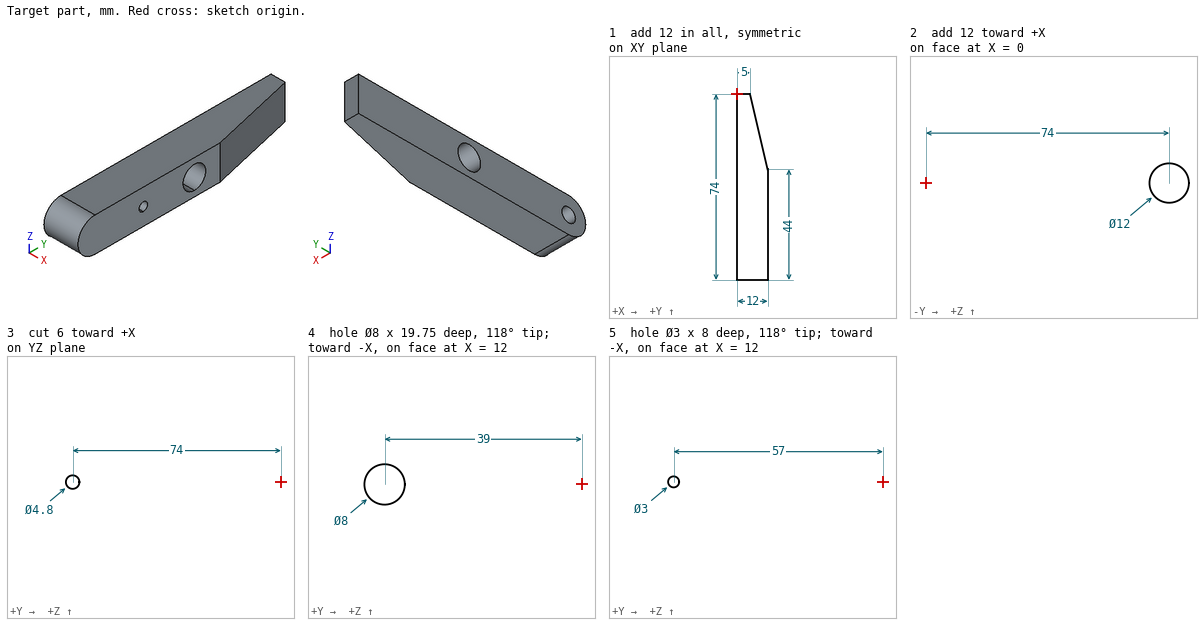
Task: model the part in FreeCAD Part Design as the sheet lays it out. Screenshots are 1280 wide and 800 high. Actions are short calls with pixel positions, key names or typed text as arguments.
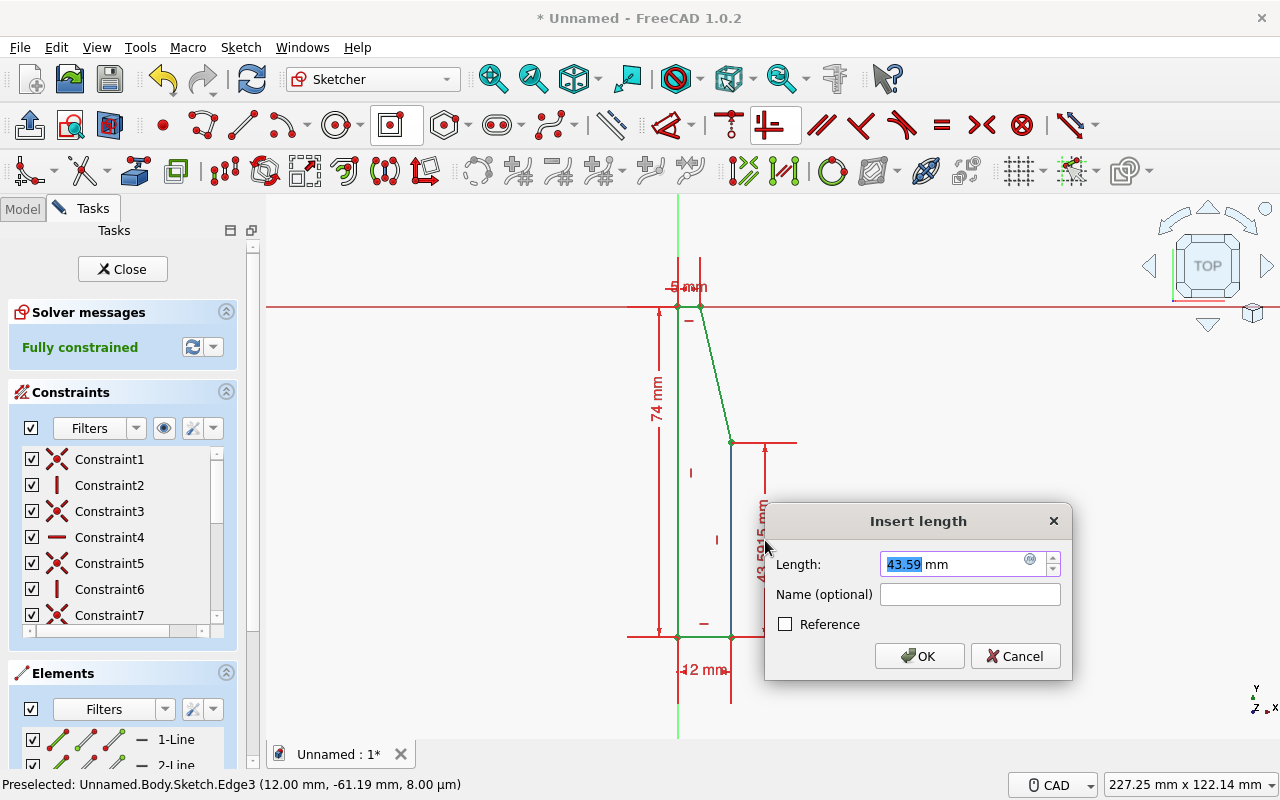
text(44)
key(Return)
key(Escape)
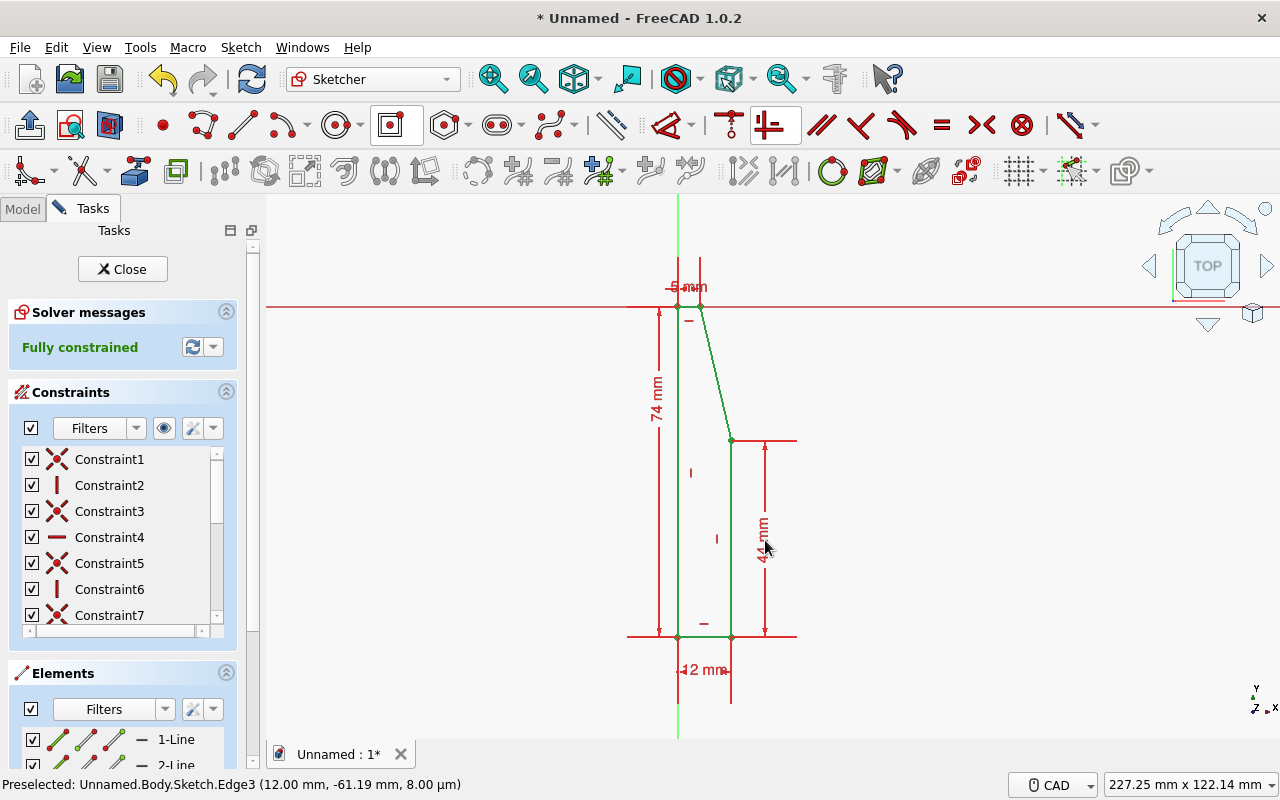
click(123, 269)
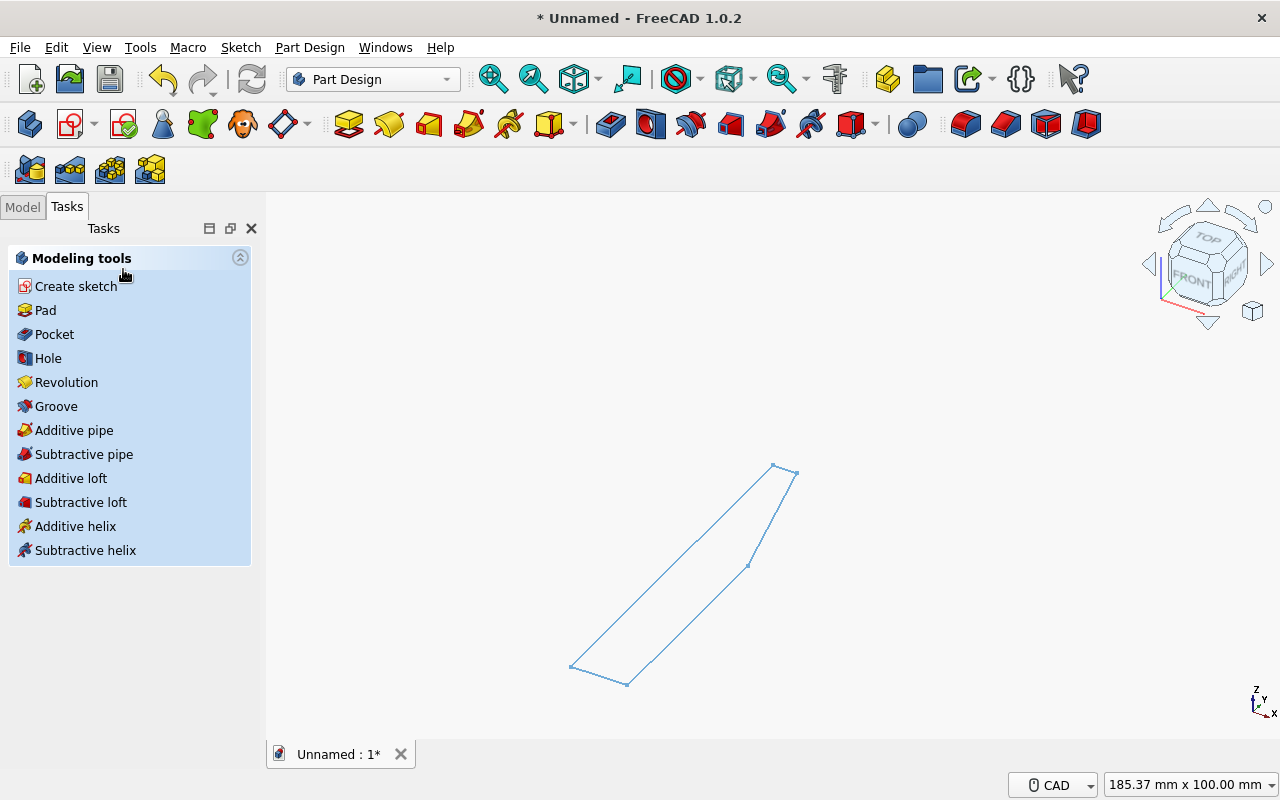
click(350, 124)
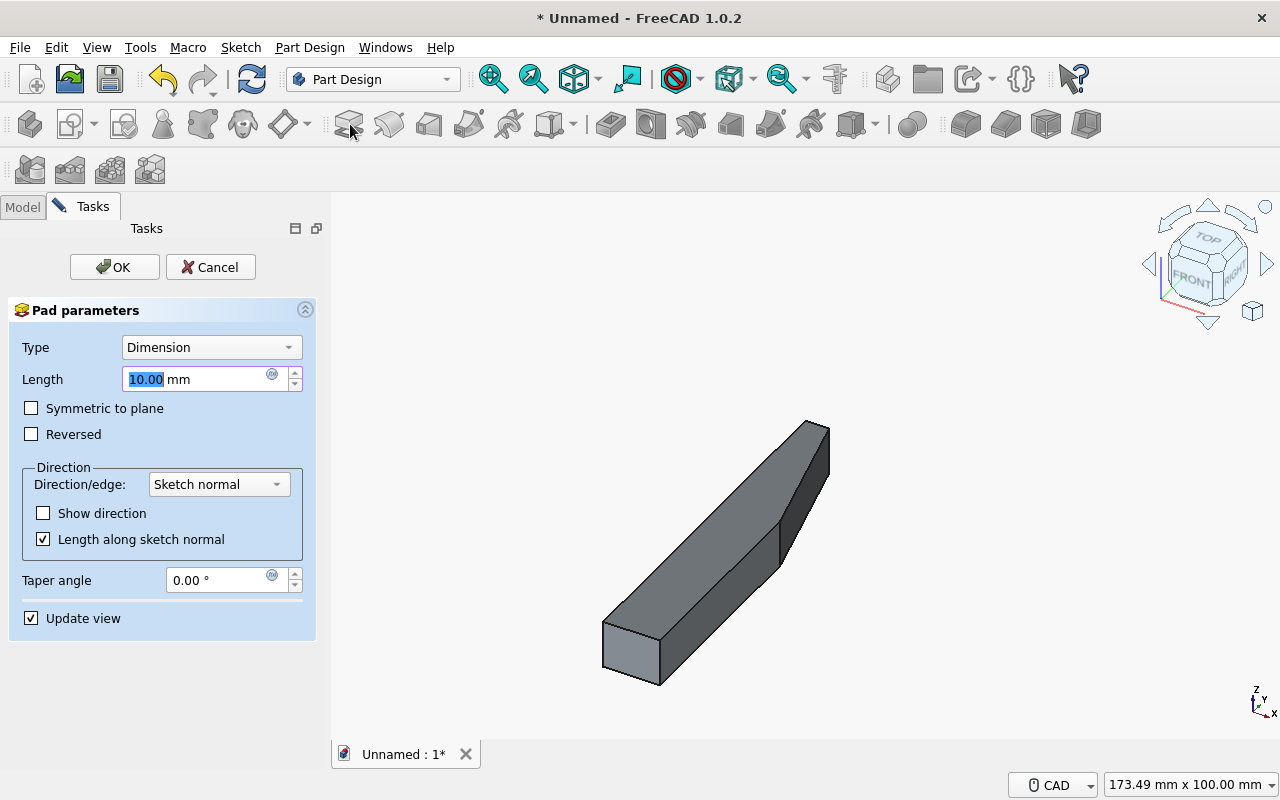
text(12)
key(Tab)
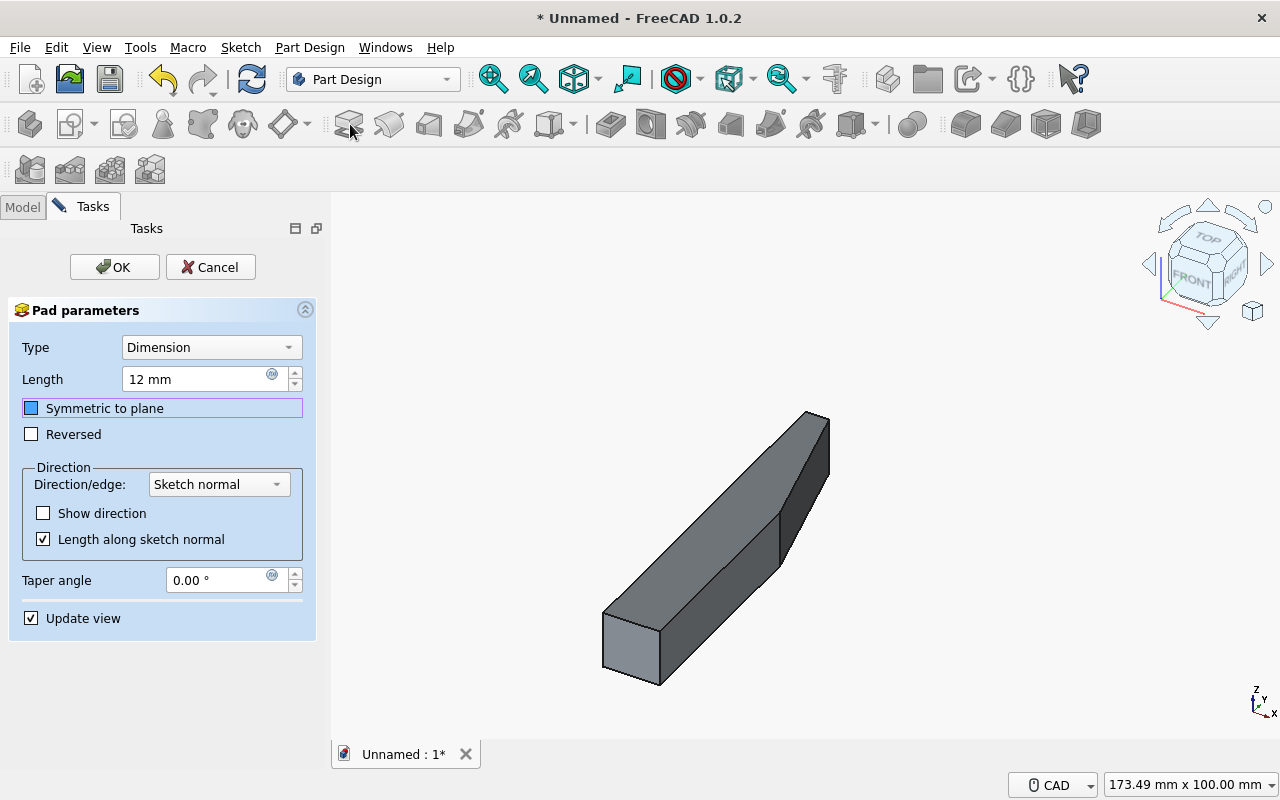
click(30, 408)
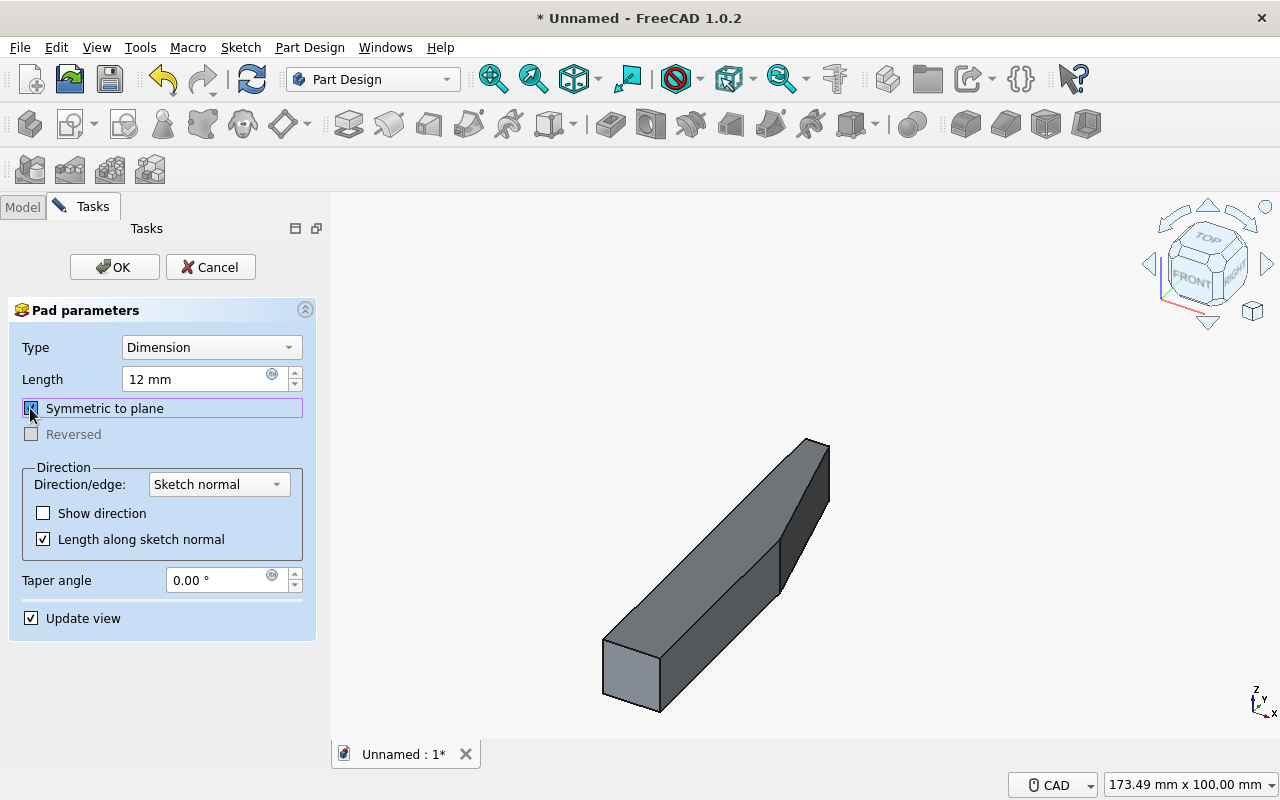
click(115, 267)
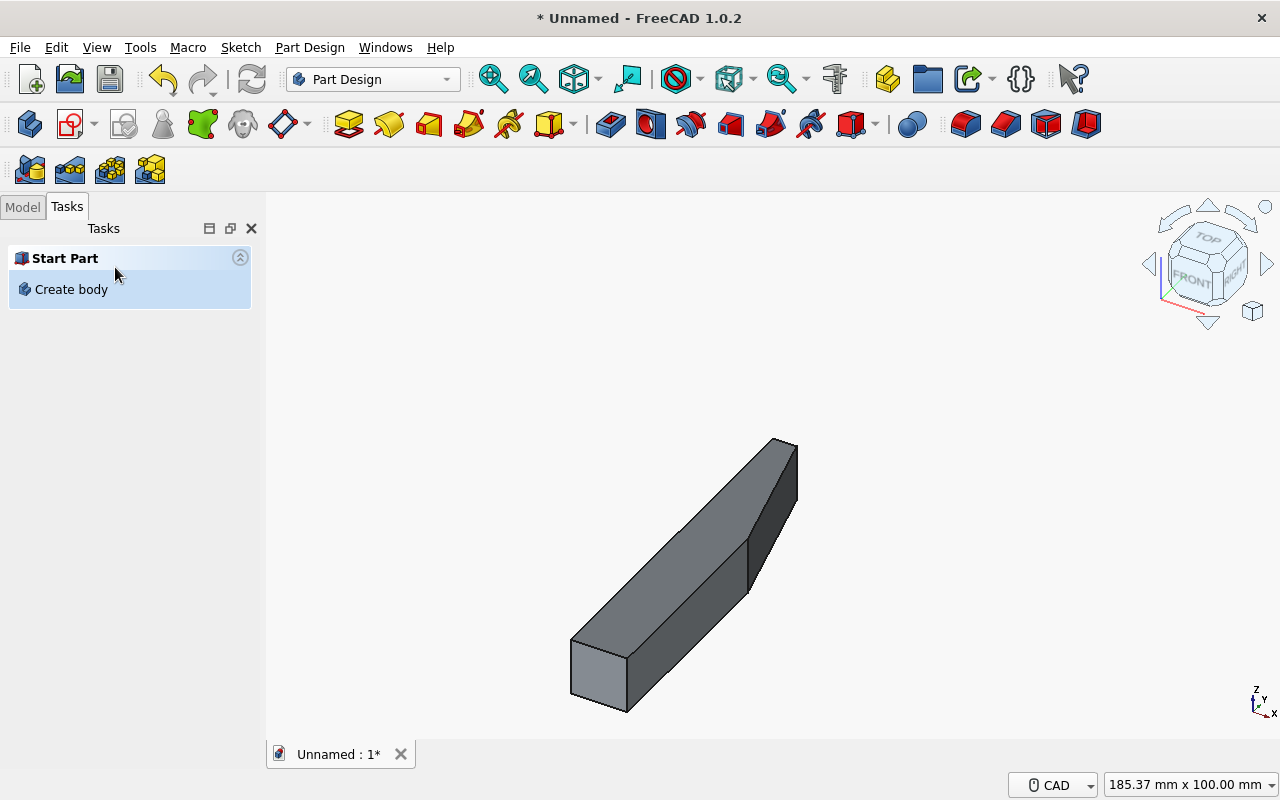
key(6)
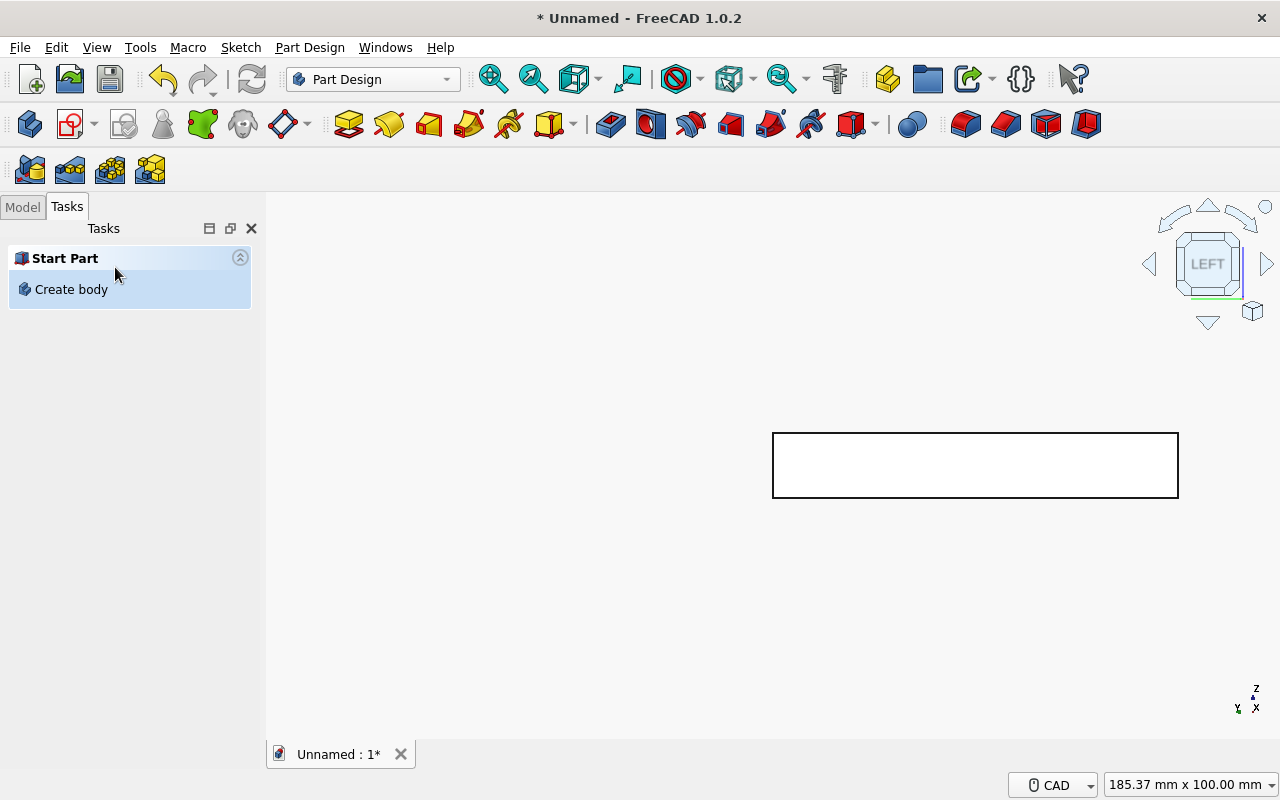
click(494, 80)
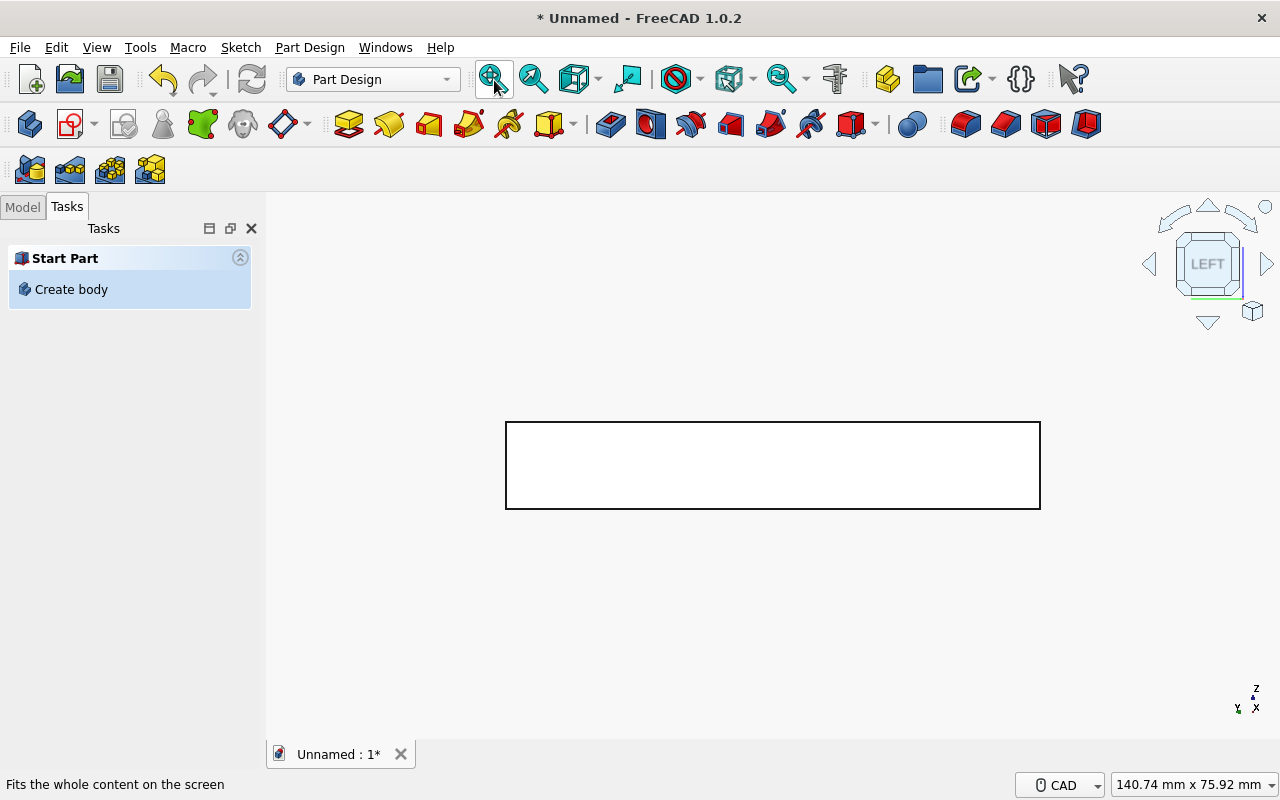
click(621, 464)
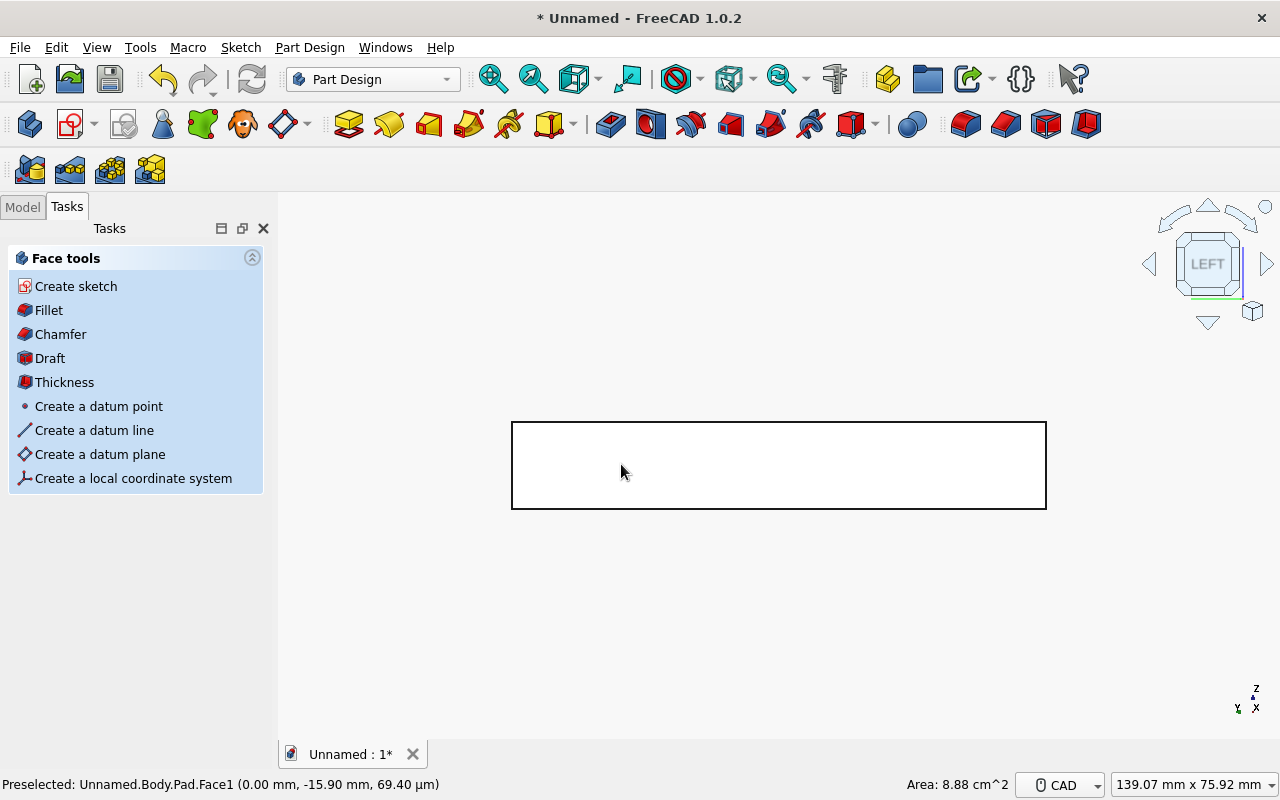
click(70, 124)